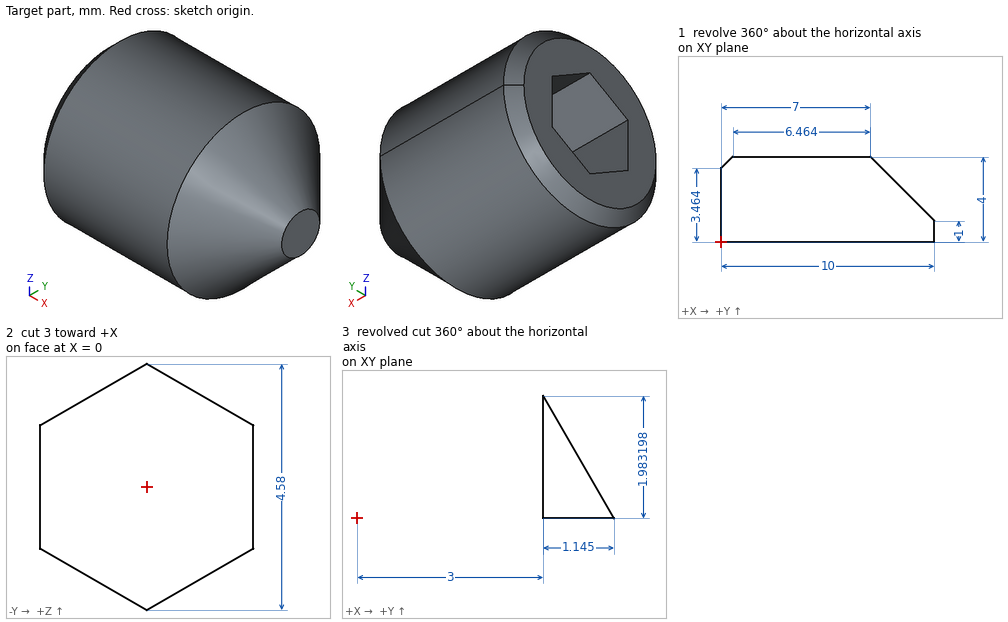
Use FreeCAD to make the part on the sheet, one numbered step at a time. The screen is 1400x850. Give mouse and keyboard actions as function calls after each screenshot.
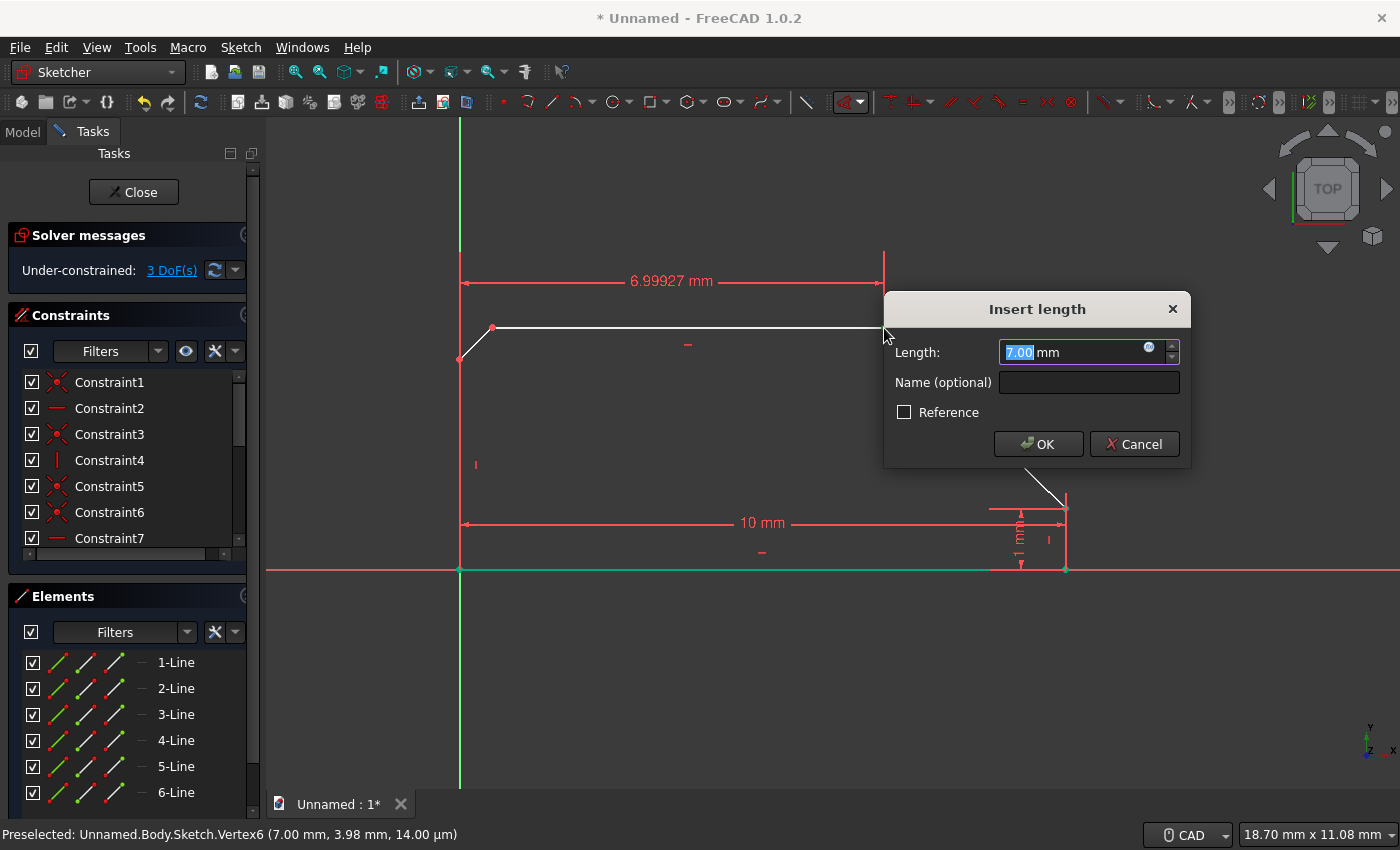
text(7)
key(Return)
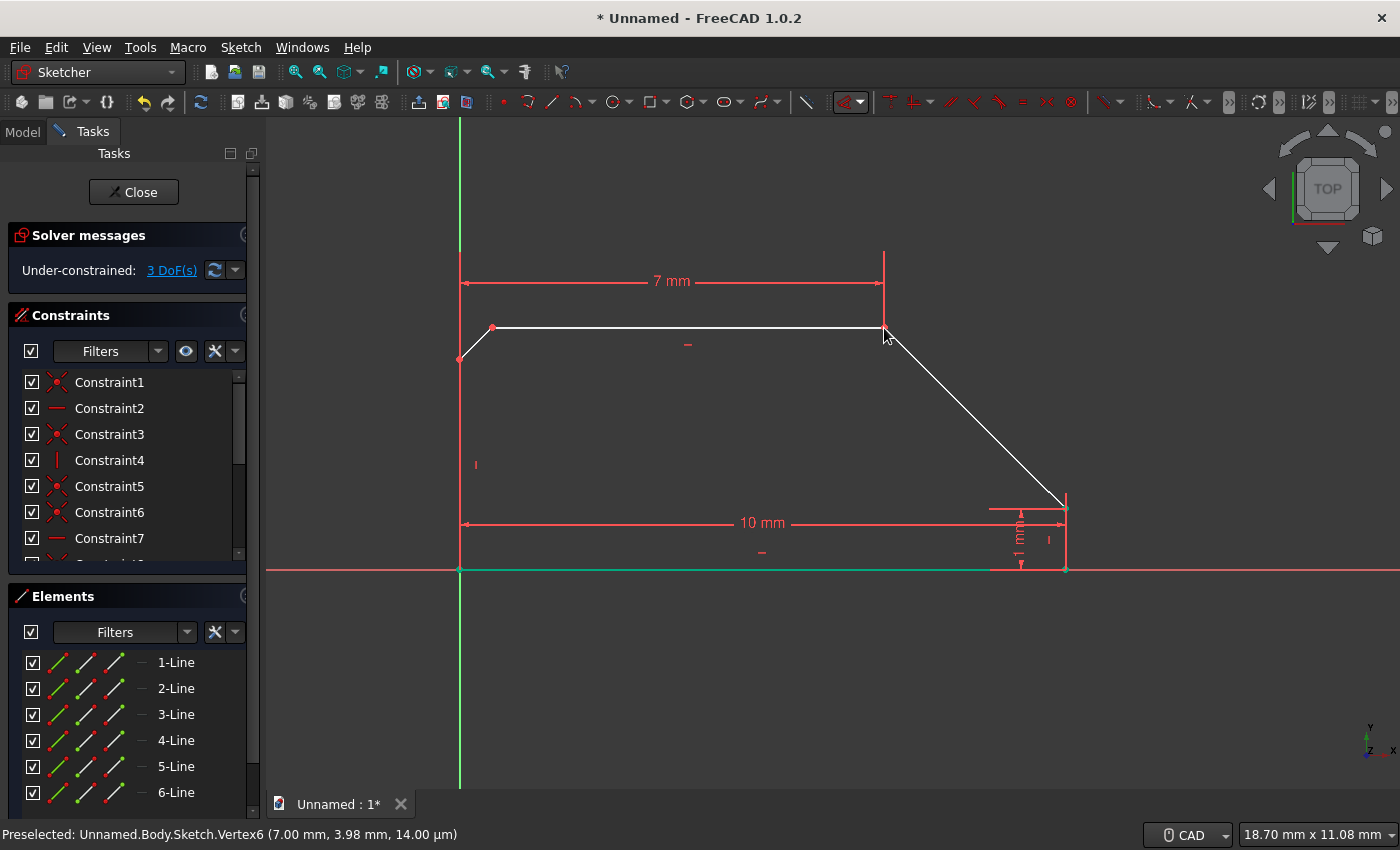
click(884, 328)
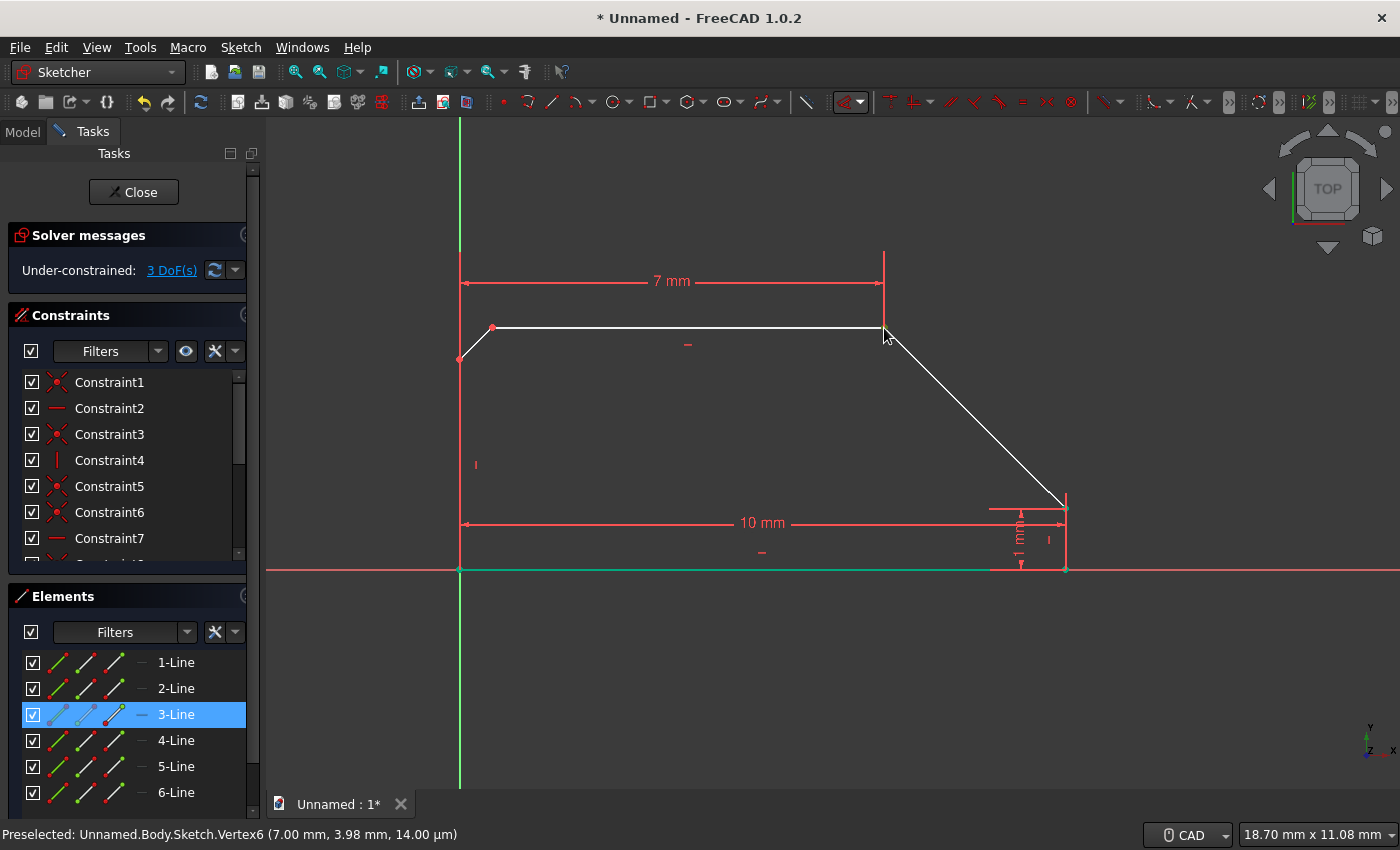
key(i)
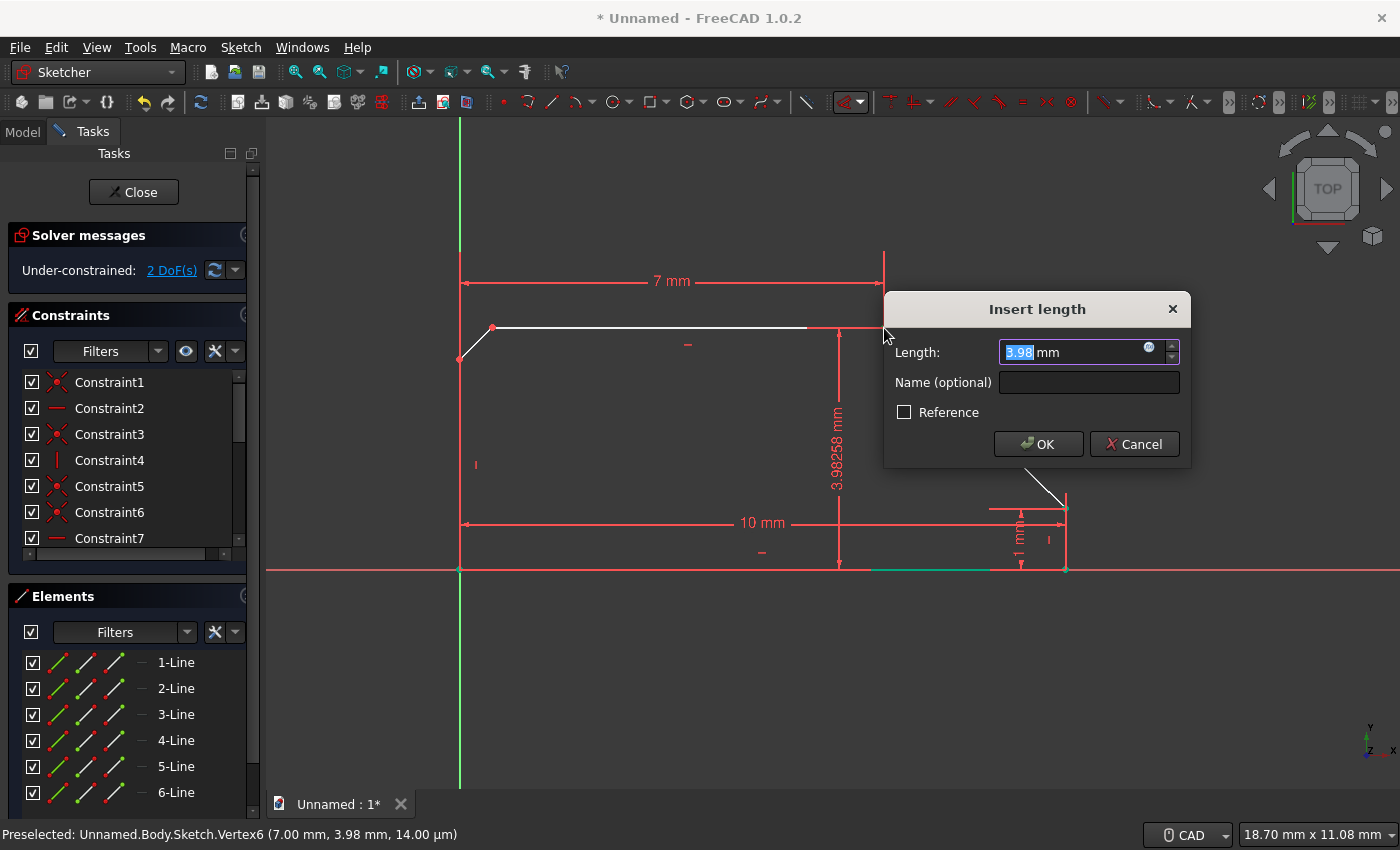
text(4)
key(Return)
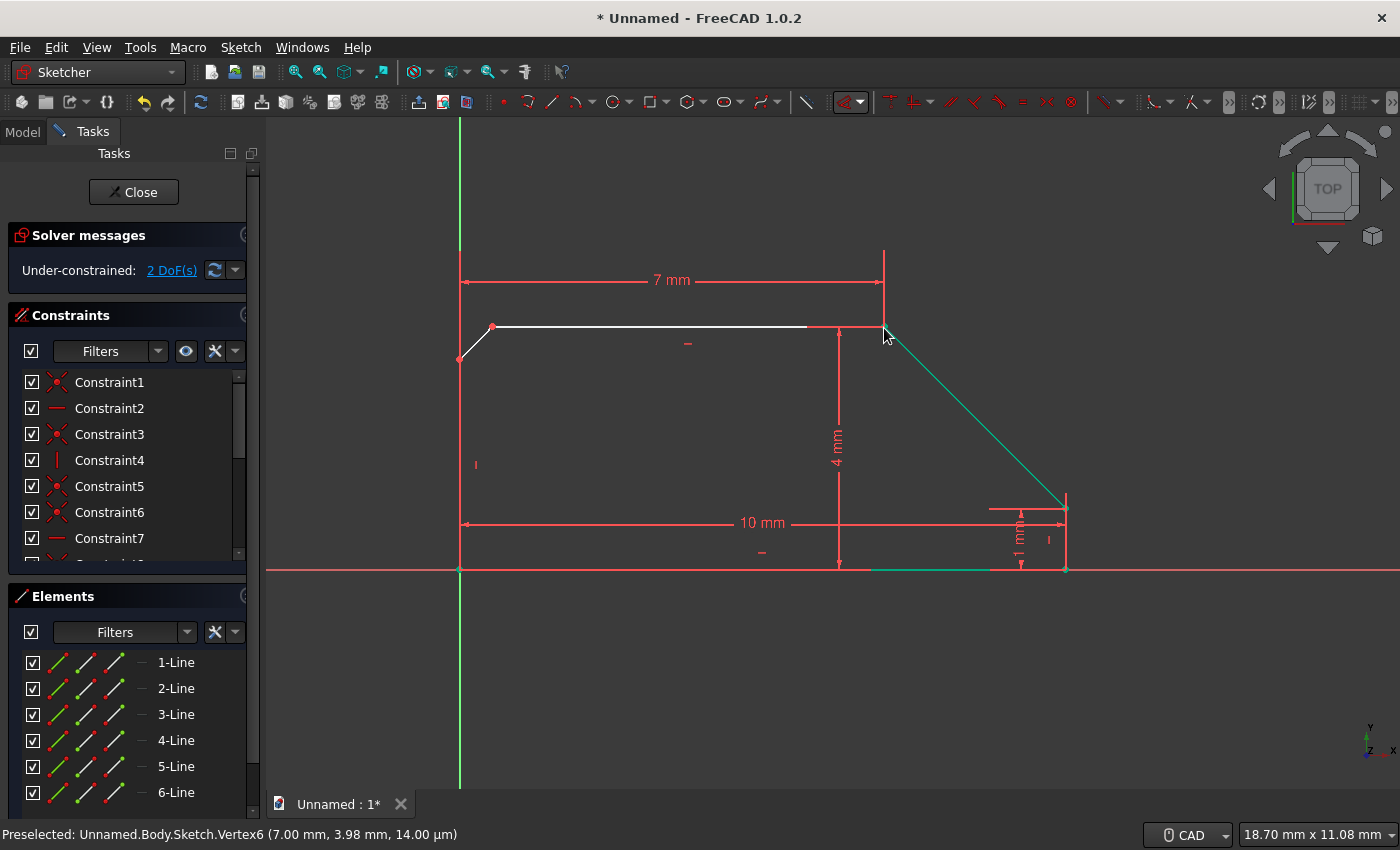
click(766, 327)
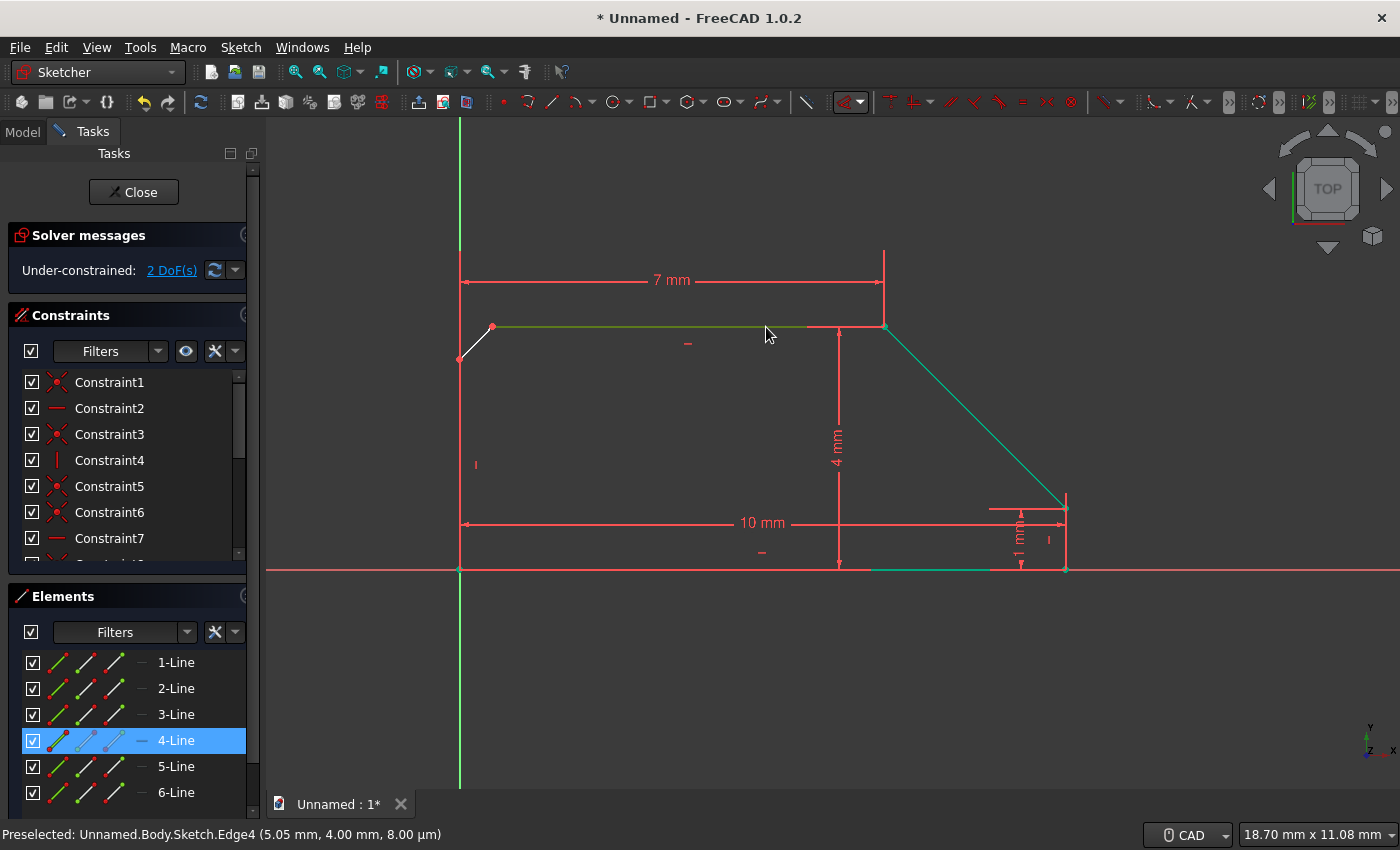
key(l)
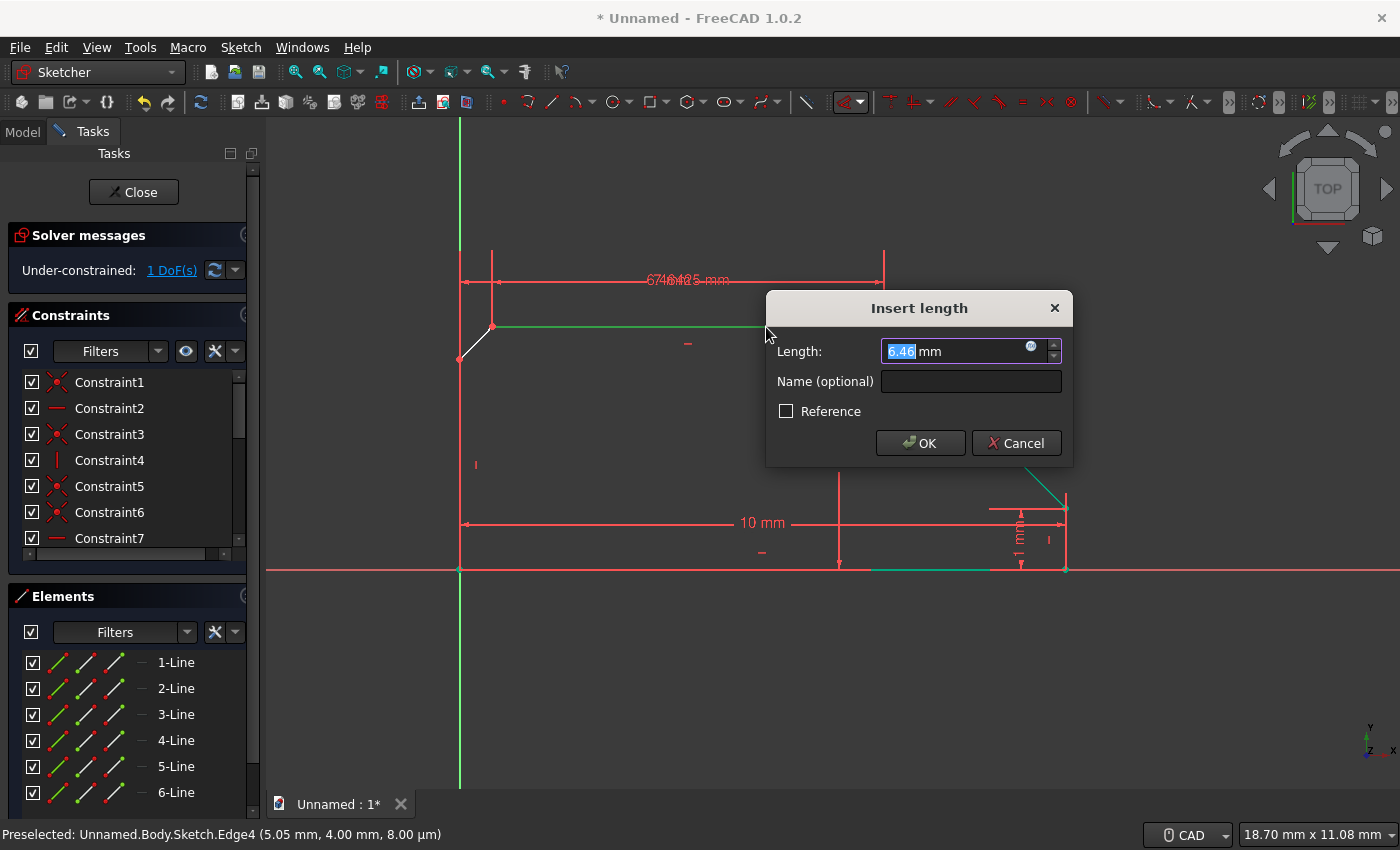
text(6.464)
key(Return)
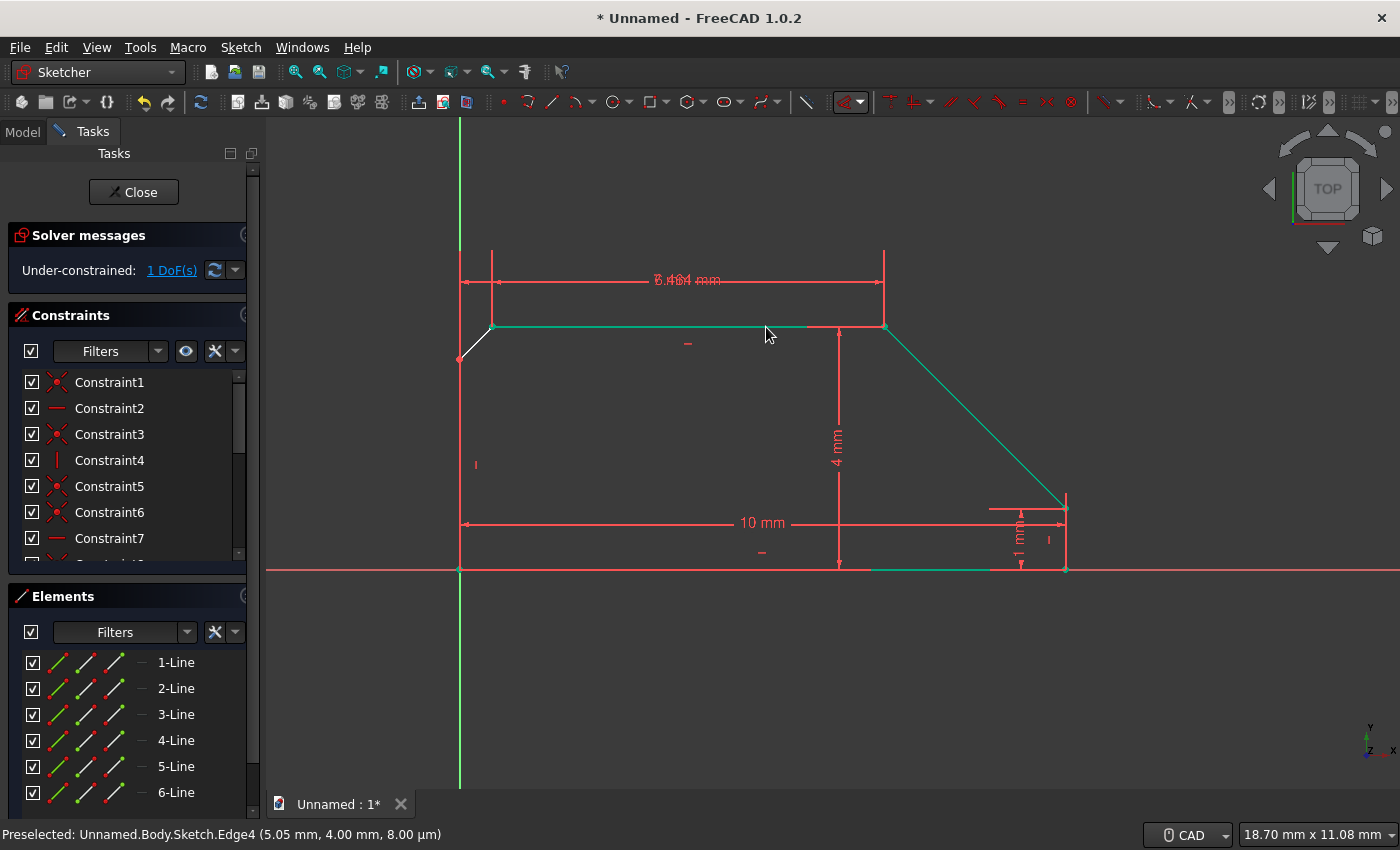
click(460, 423)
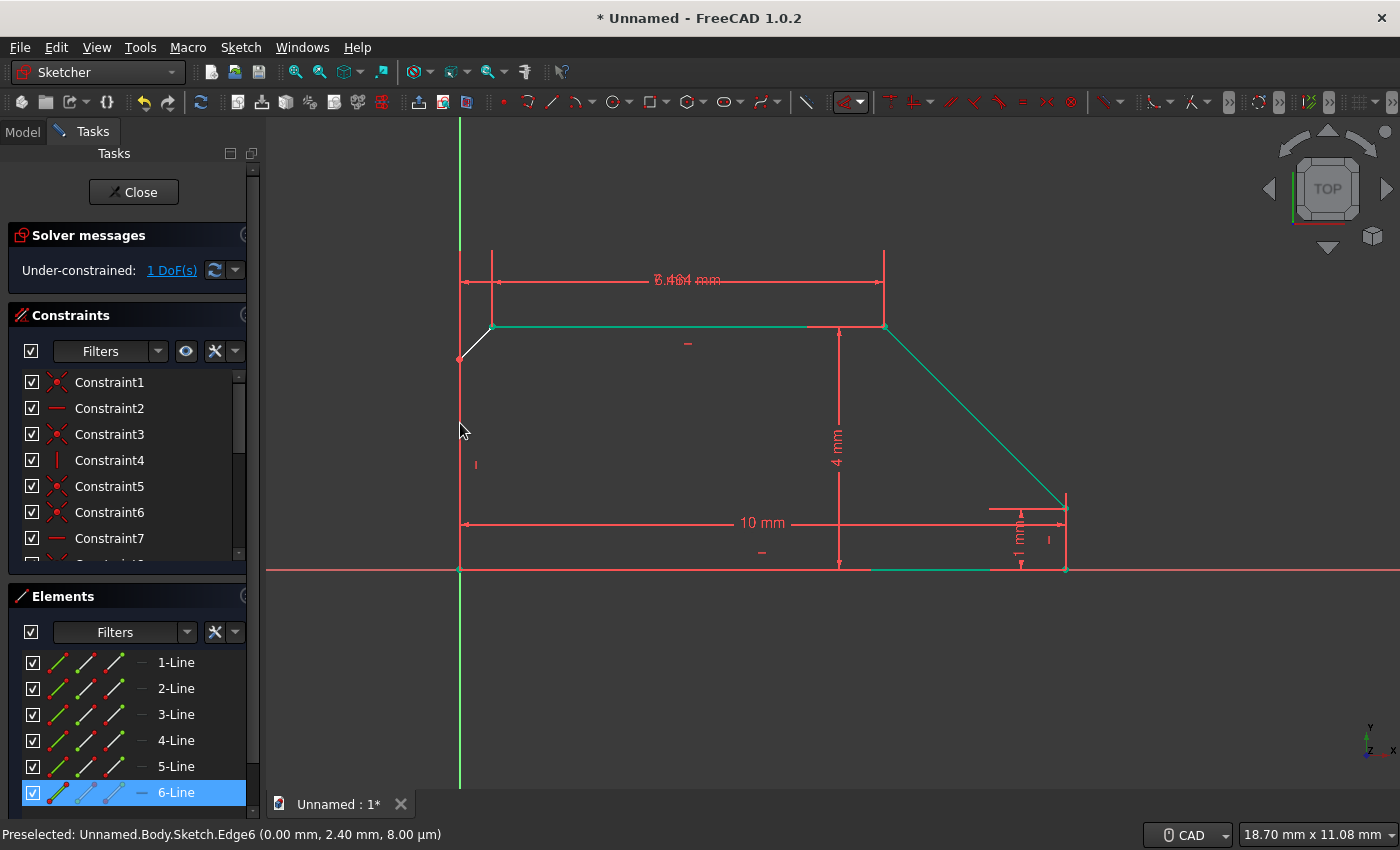
key(i)